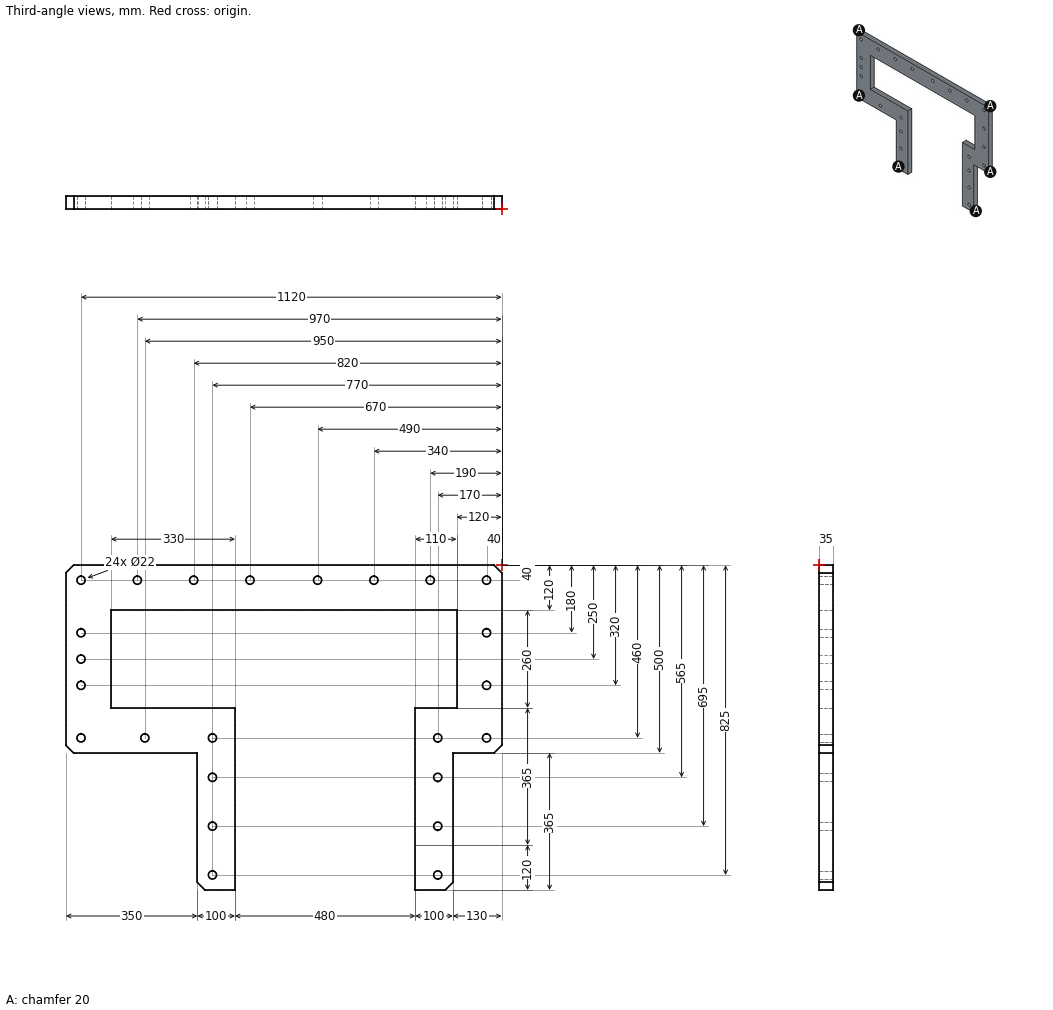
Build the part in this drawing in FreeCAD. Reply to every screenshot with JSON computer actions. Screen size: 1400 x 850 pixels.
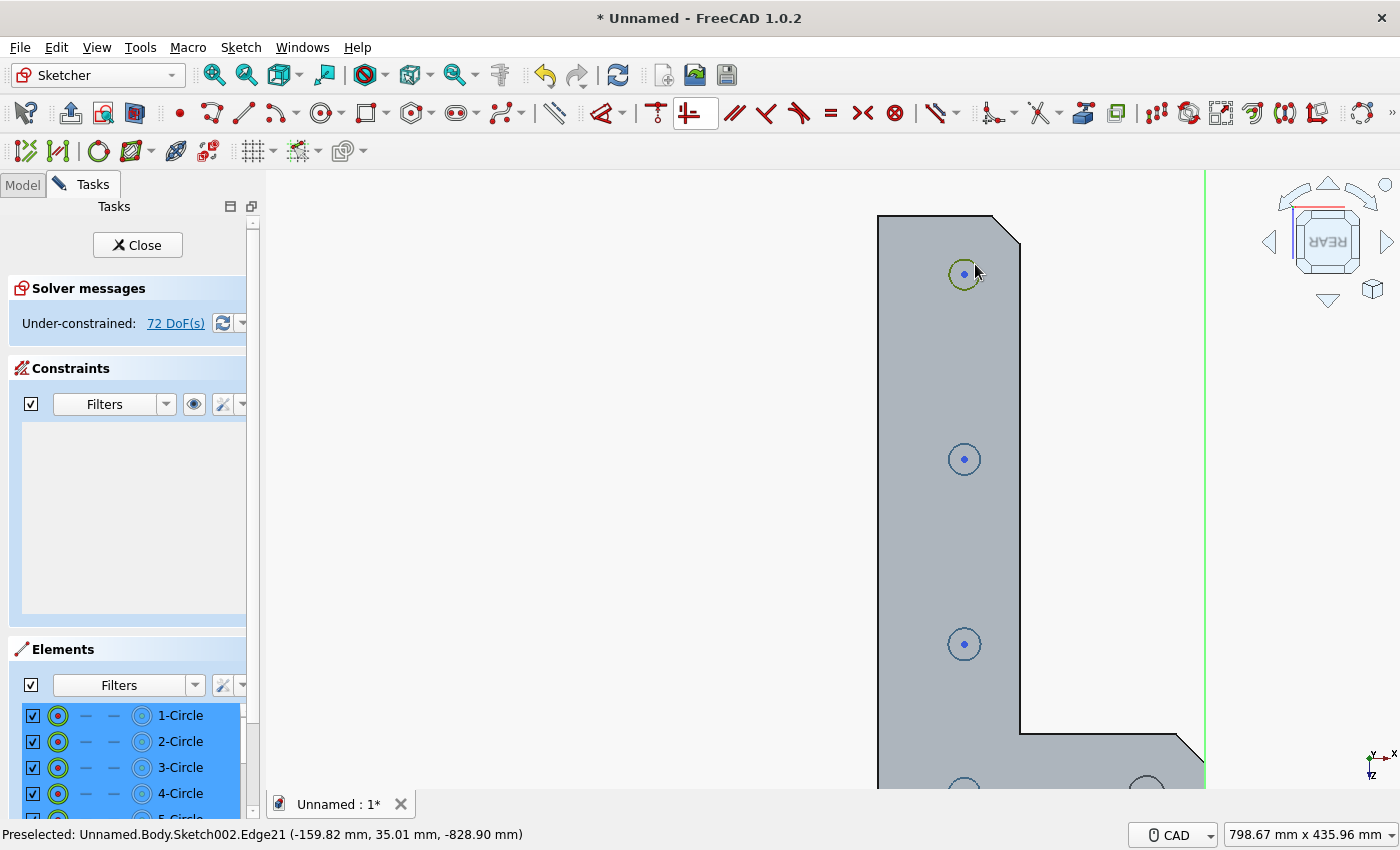
{"action": "scroll", "coordinate": [976, 263], "scroll_direction": "down", "scroll_amount": 5}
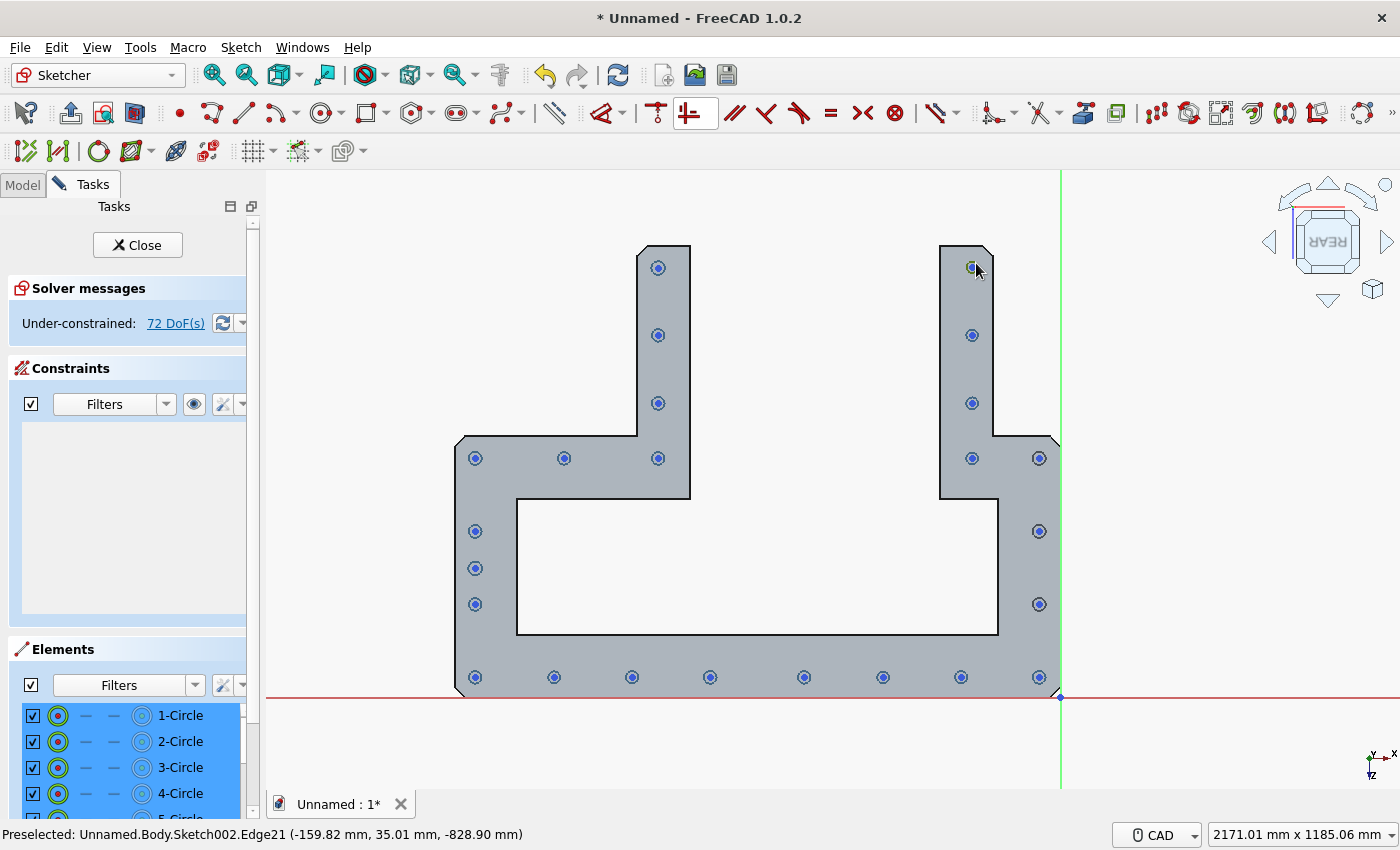
{"action": "scroll", "coordinate": [1044, 454], "scroll_direction": "up", "scroll_amount": 4}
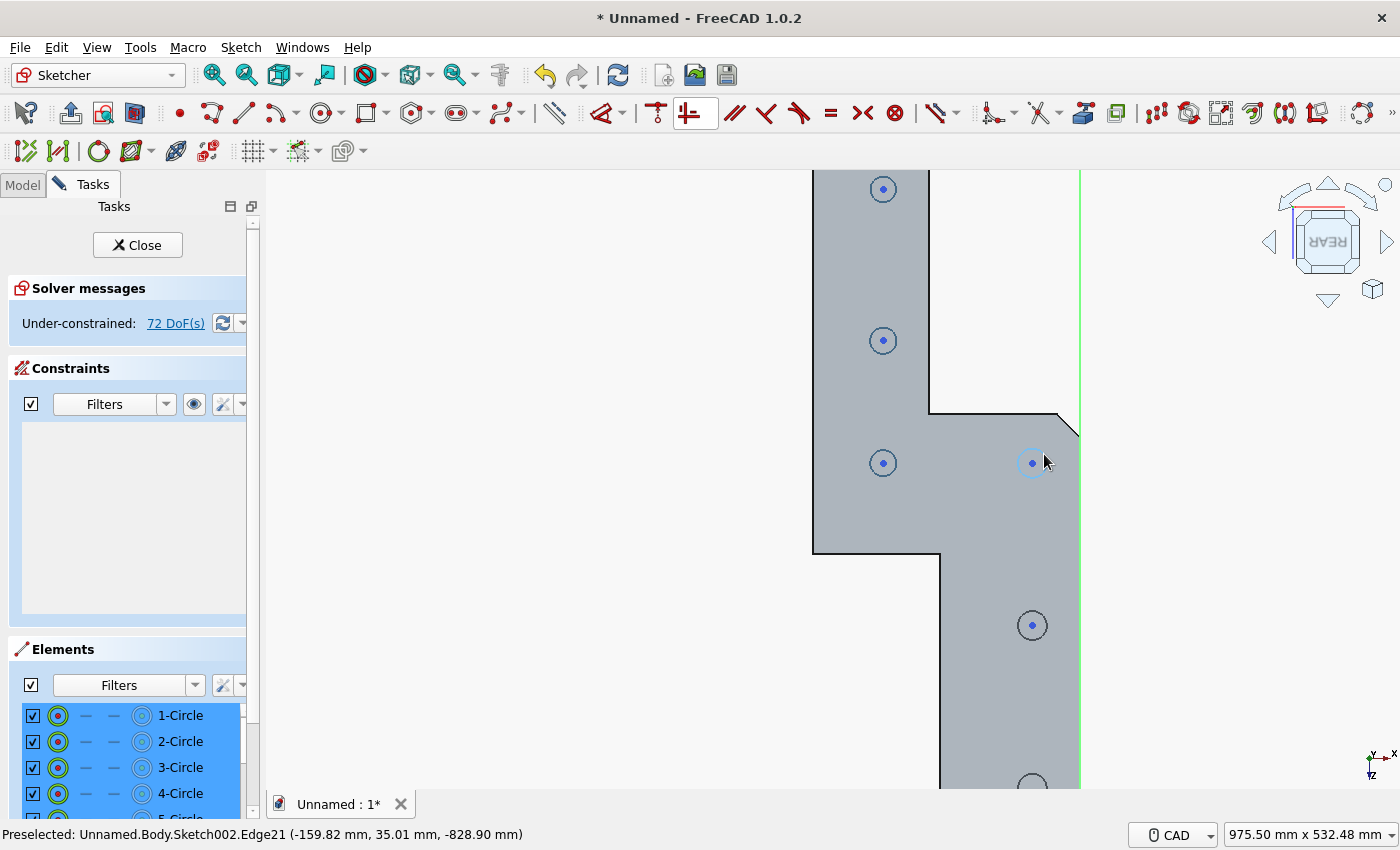
{"action": "left_click", "coordinate": [1043, 453]}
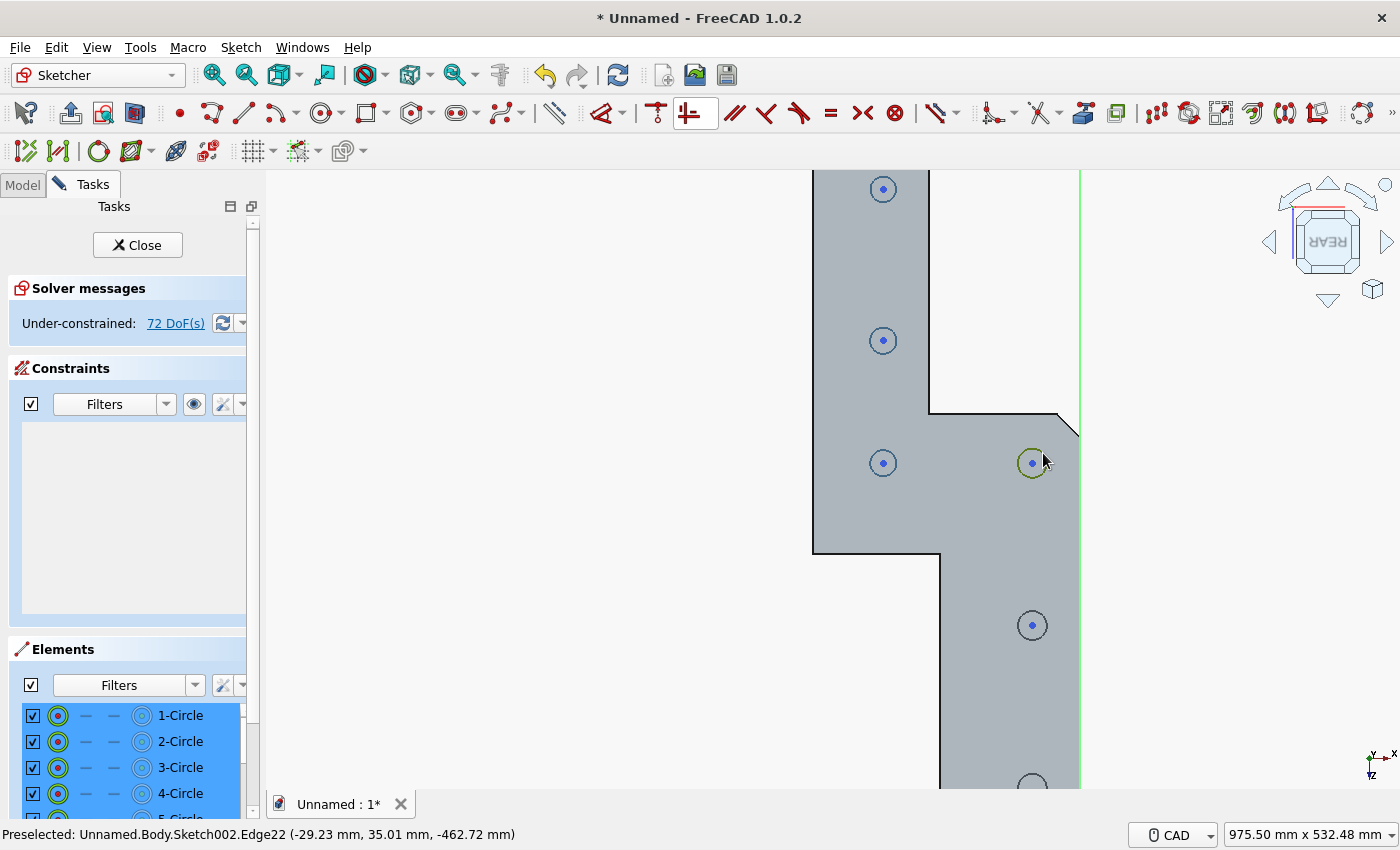
{"action": "left_click", "coordinate": [1043, 615]}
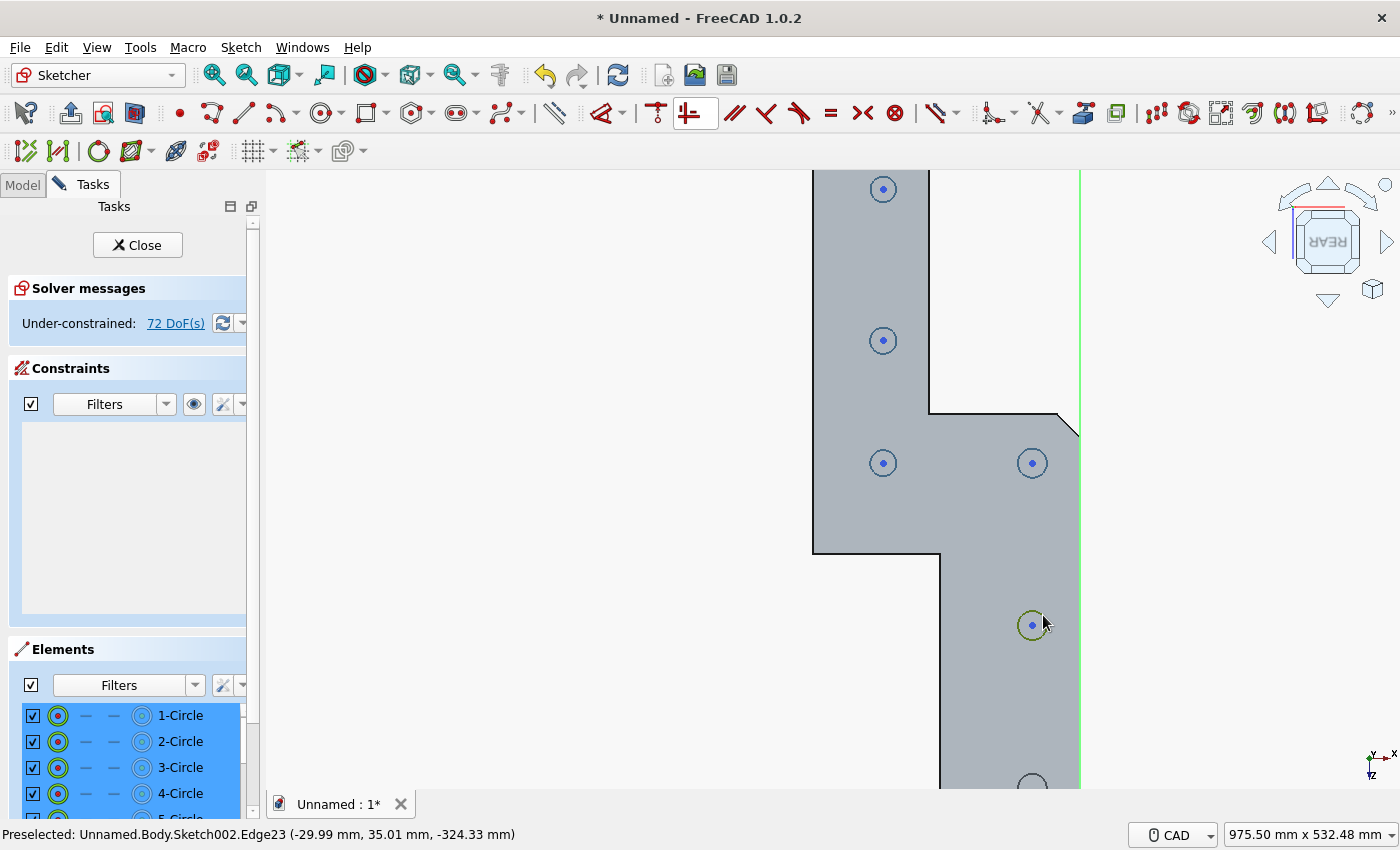
{"action": "scroll", "coordinate": [1044, 455], "scroll_direction": "down", "scroll_amount": 4}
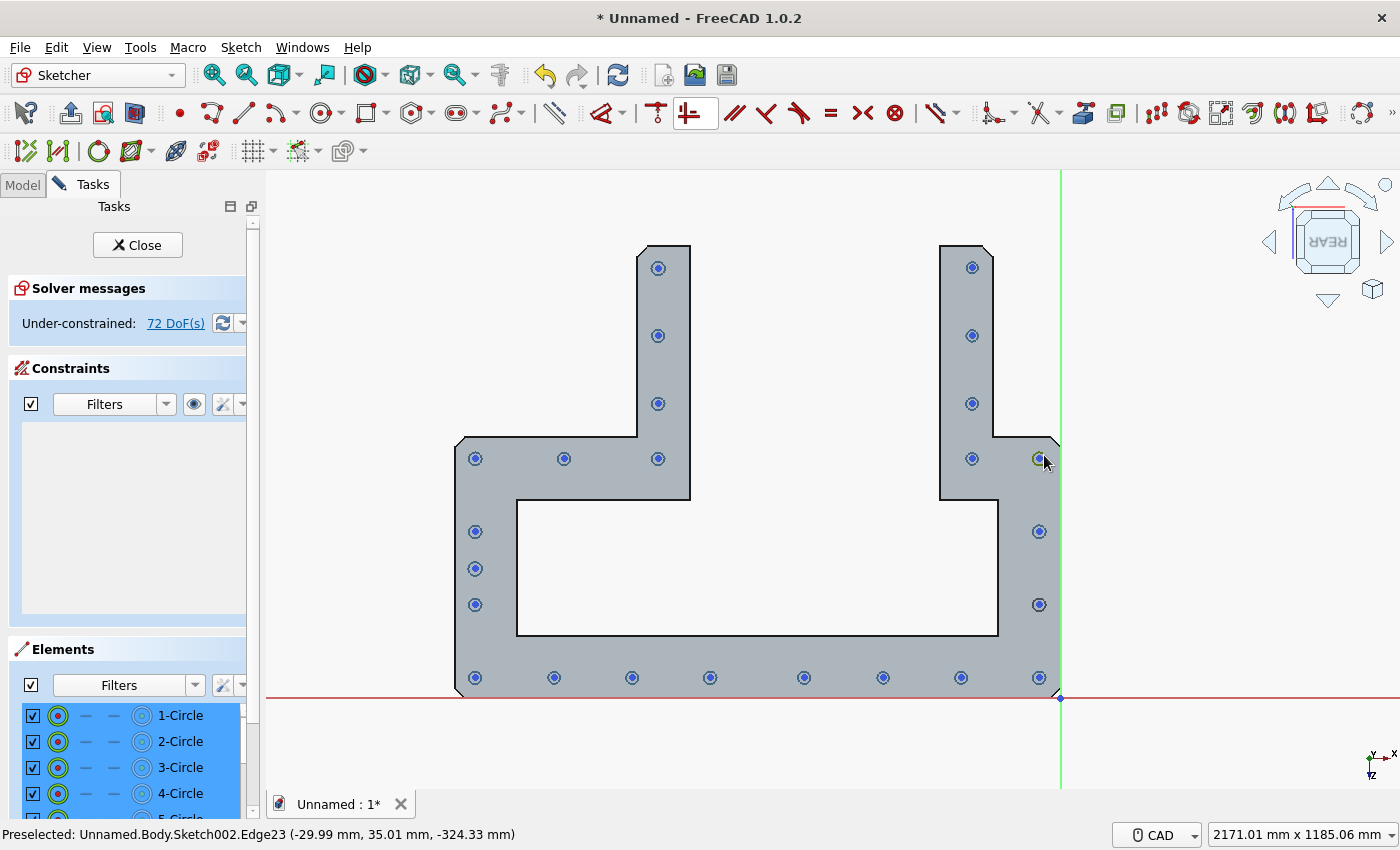
{"action": "scroll", "coordinate": [1044, 600], "scroll_direction": "up", "scroll_amount": 4}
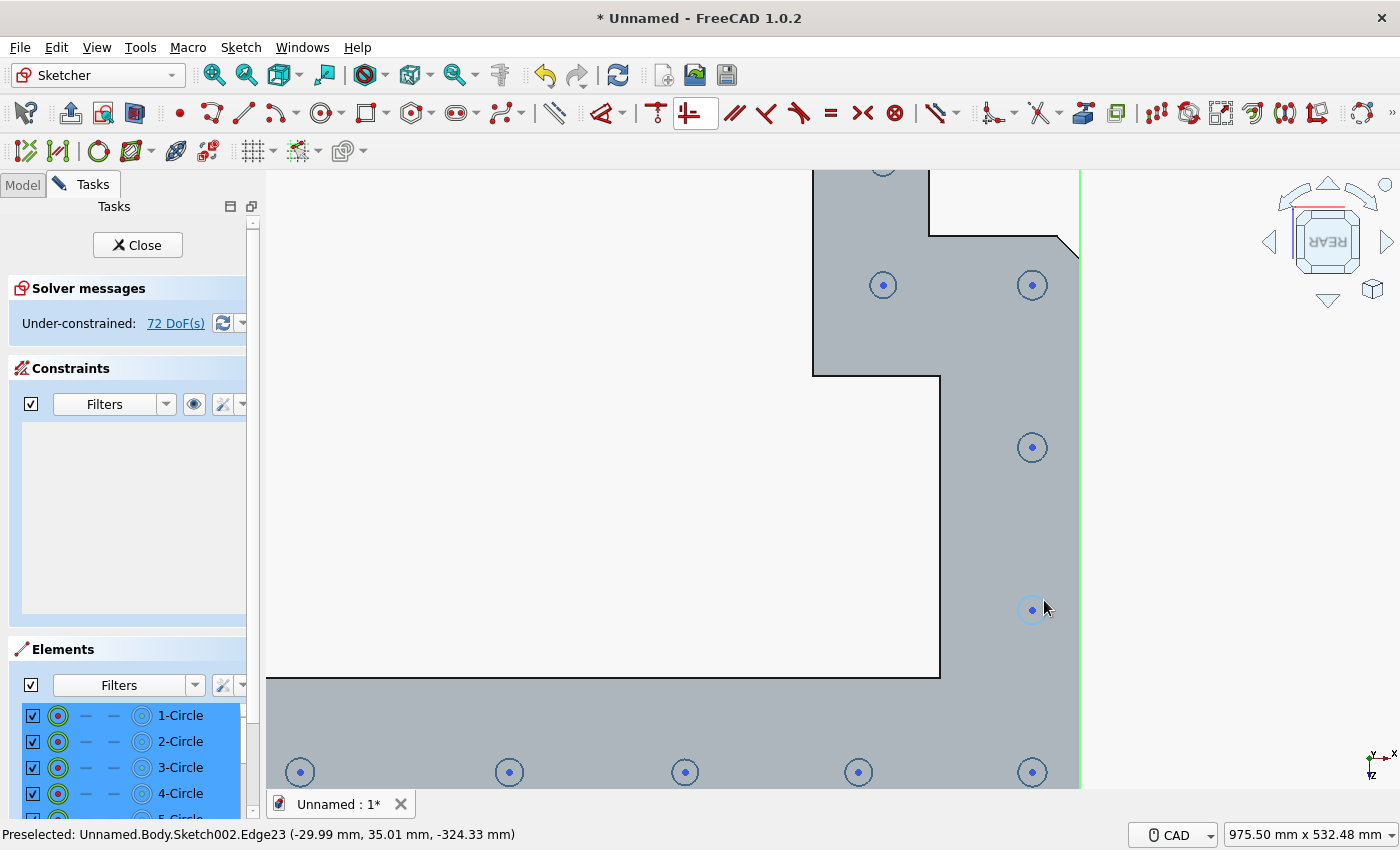
{"action": "left_click", "coordinate": [1042, 600]}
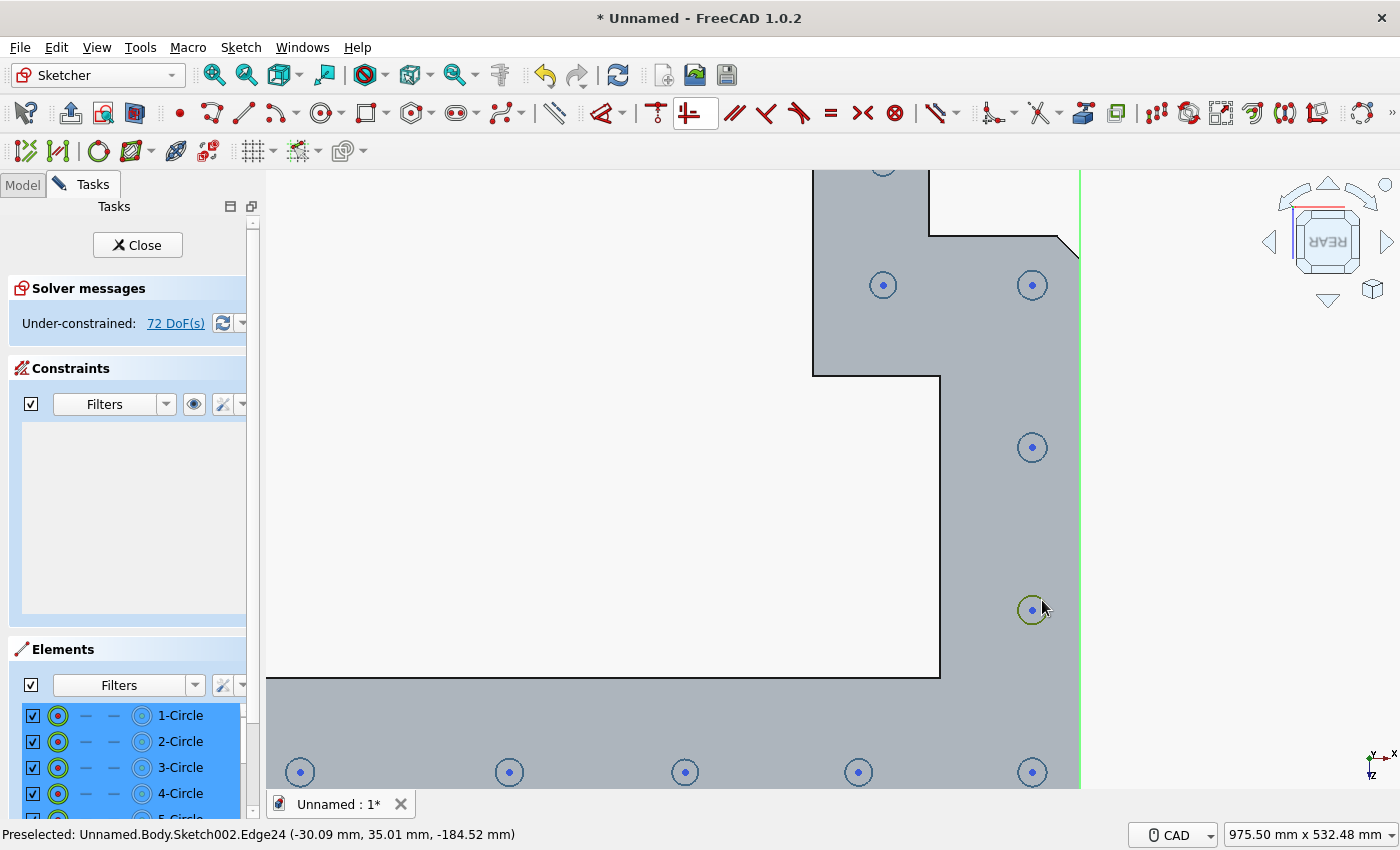
{"action": "key", "text": "e"}